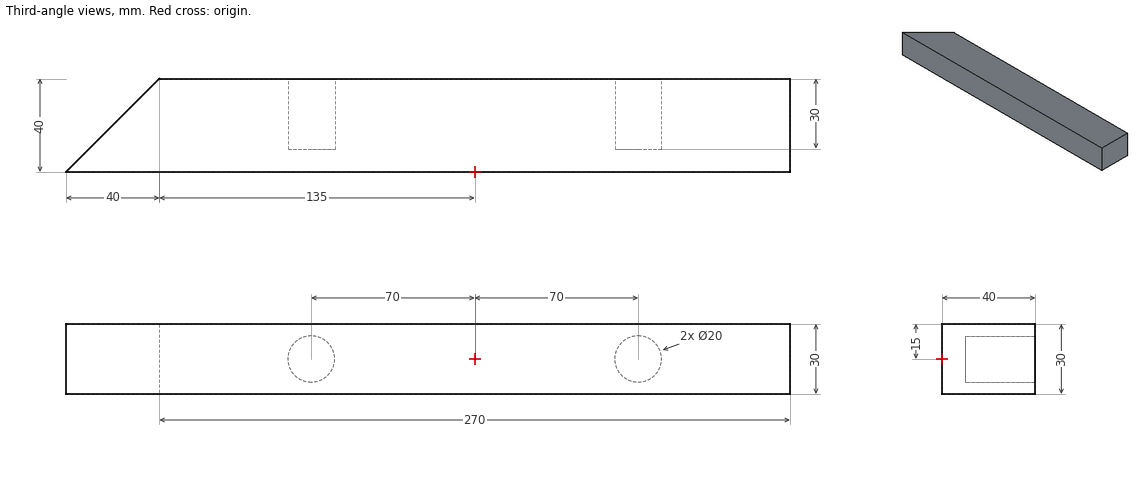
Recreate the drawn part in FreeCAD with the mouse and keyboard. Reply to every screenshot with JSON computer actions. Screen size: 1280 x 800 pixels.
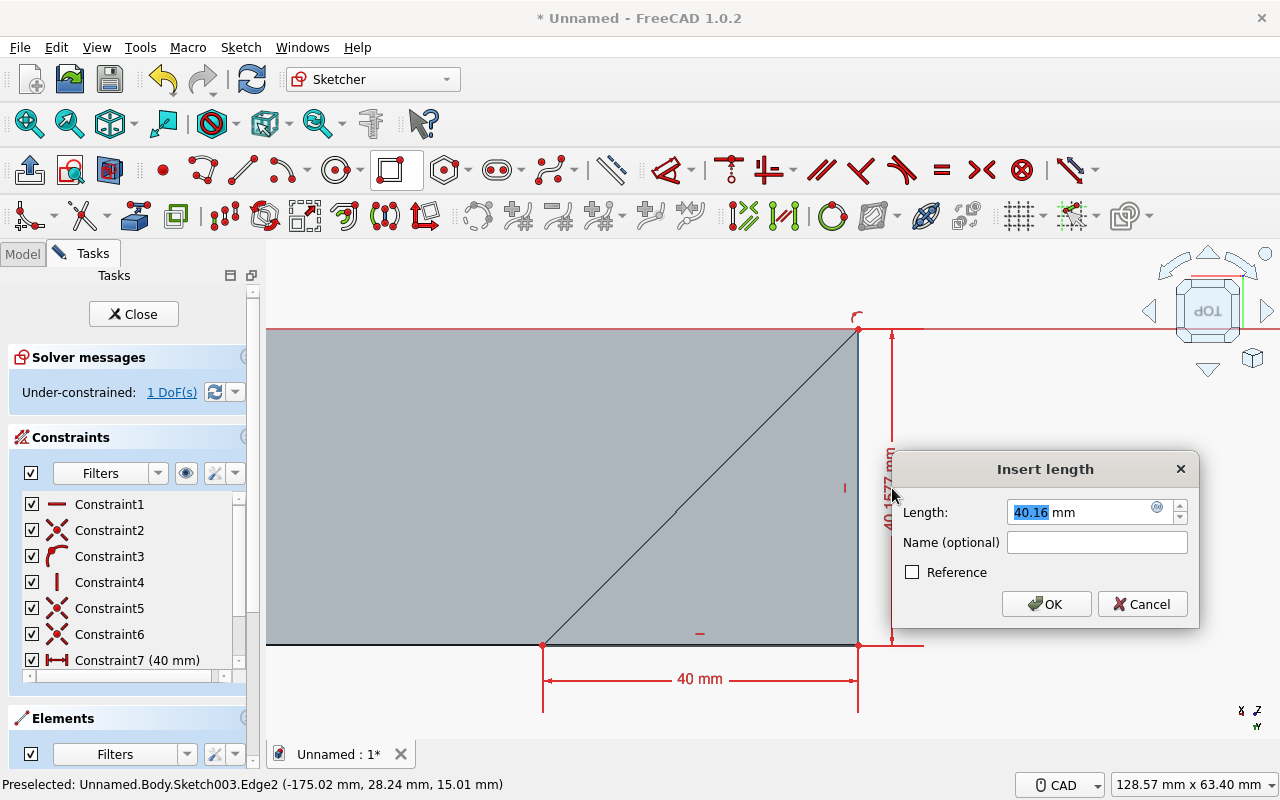
{"action": "type", "text": "40"}
{"action": "key", "text": "Return"}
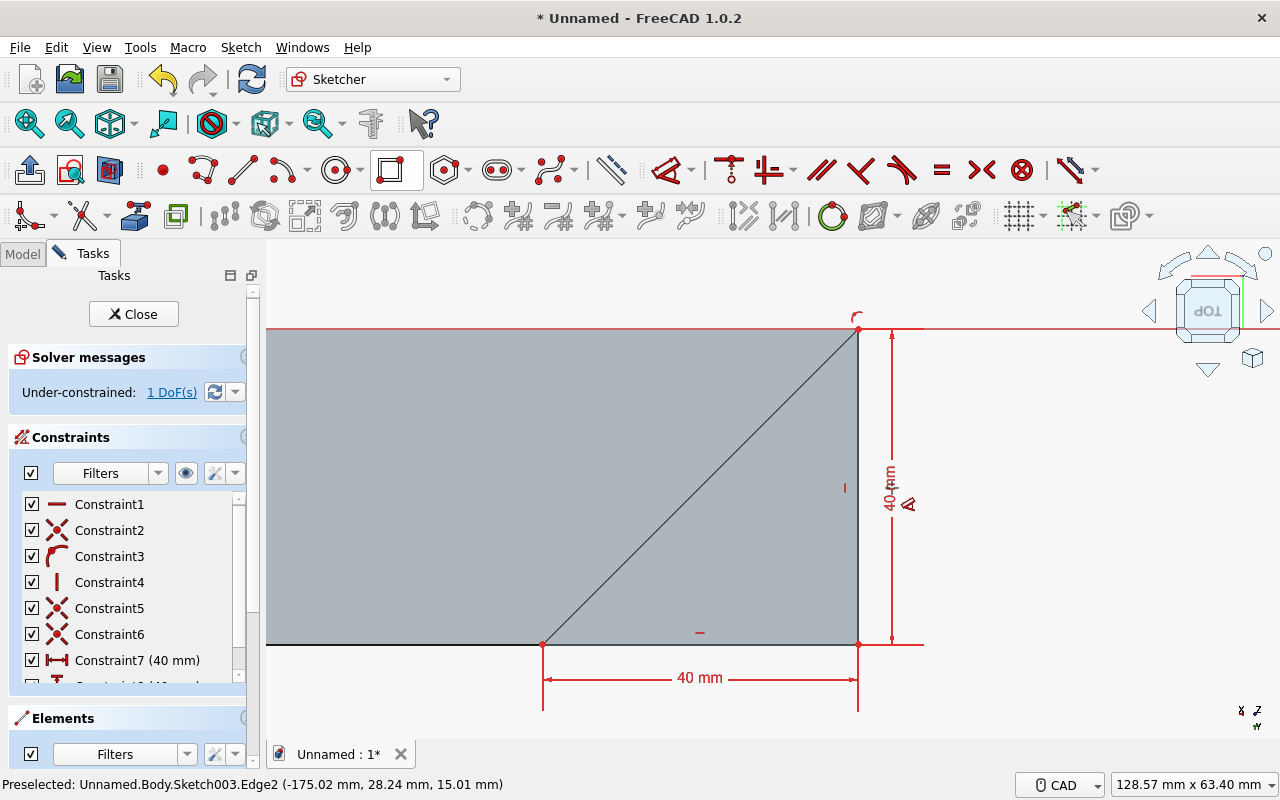
{"action": "left_click", "coordinate": [543, 645]}
{"action": "left_click", "coordinate": [418, 679]}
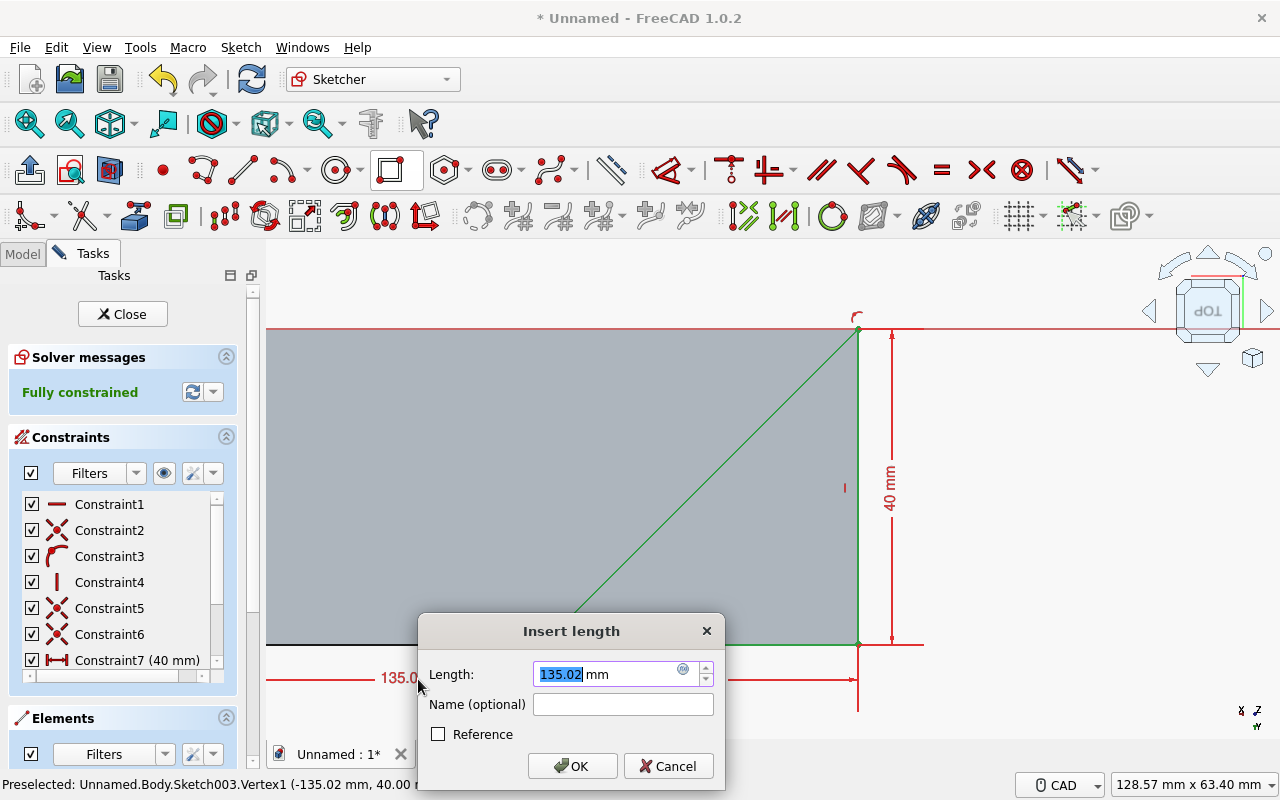
{"action": "type", "text": "135"}
{"action": "key", "text": "Return"}
{"action": "key", "text": "Escape"}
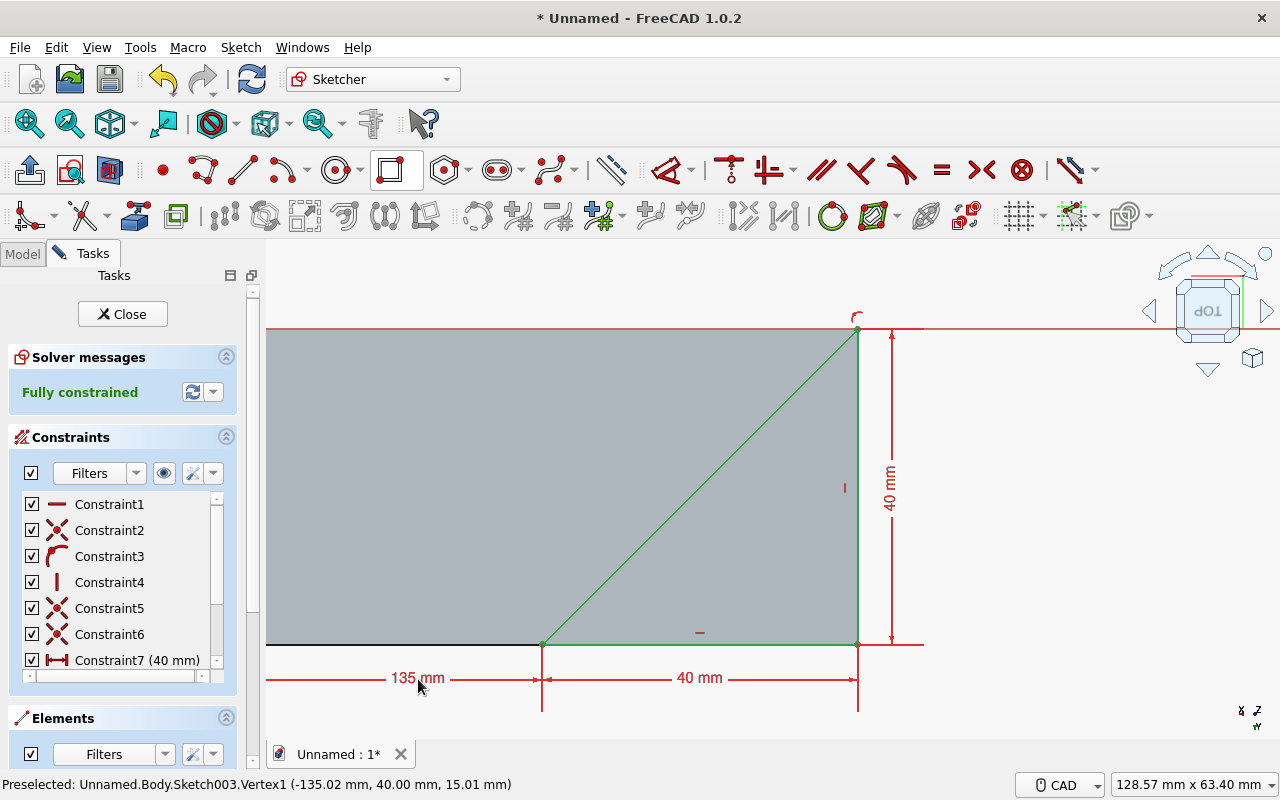
{"action": "left_click", "coordinate": [123, 314]}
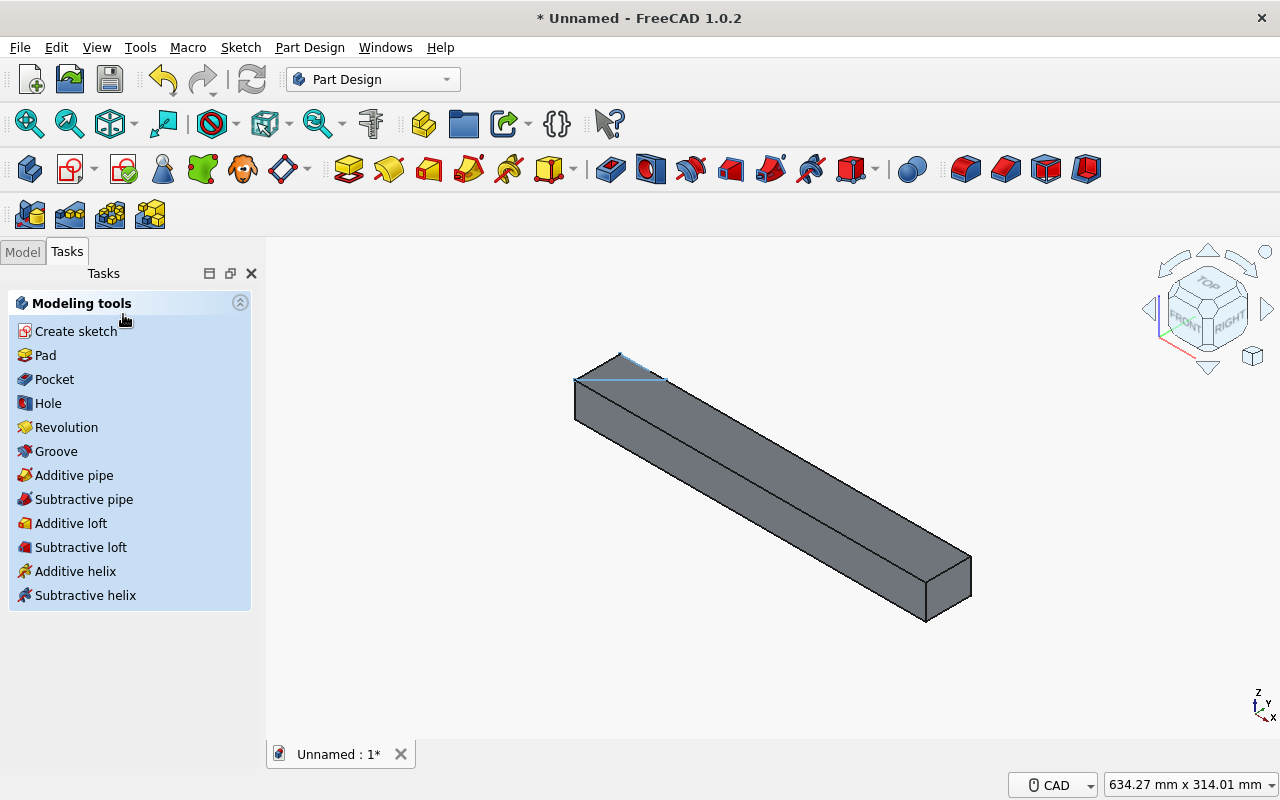
{"action": "left_click", "coordinate": [612, 170]}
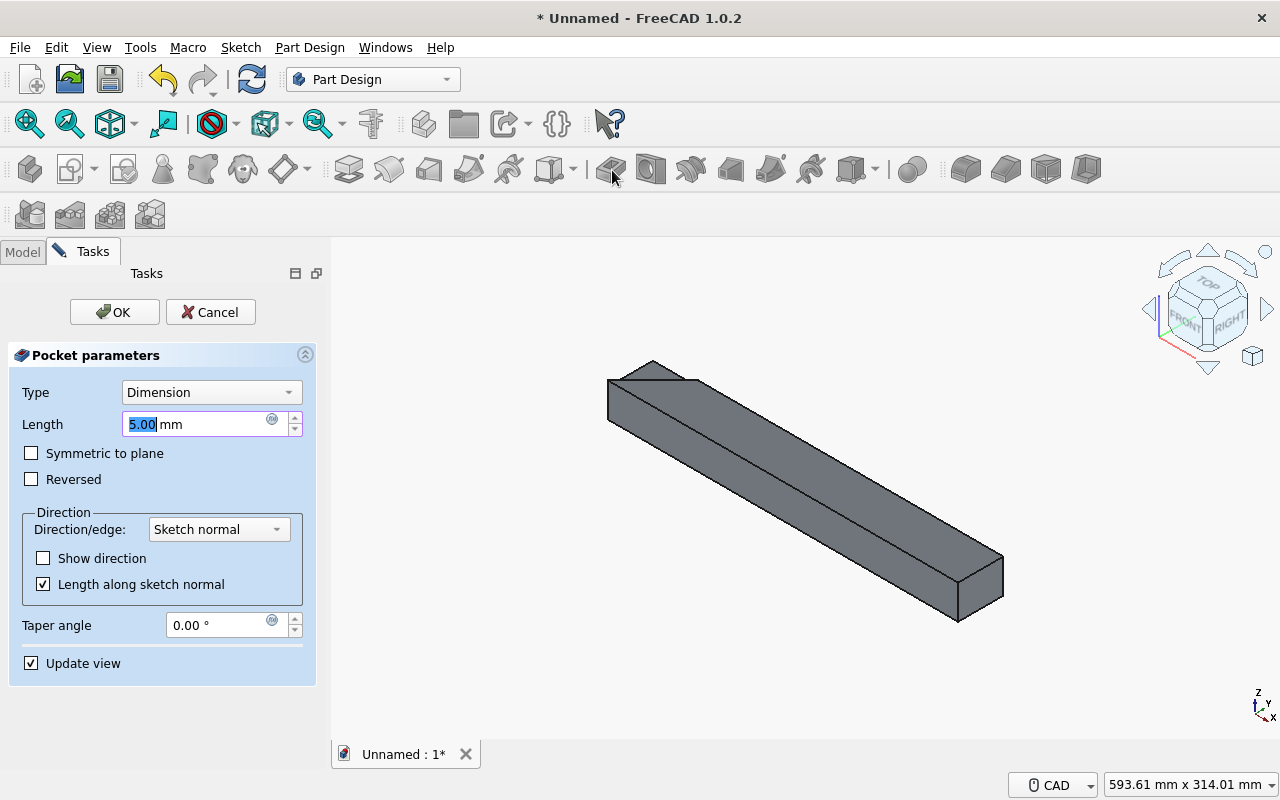
{"action": "left_click", "coordinate": [212, 392]}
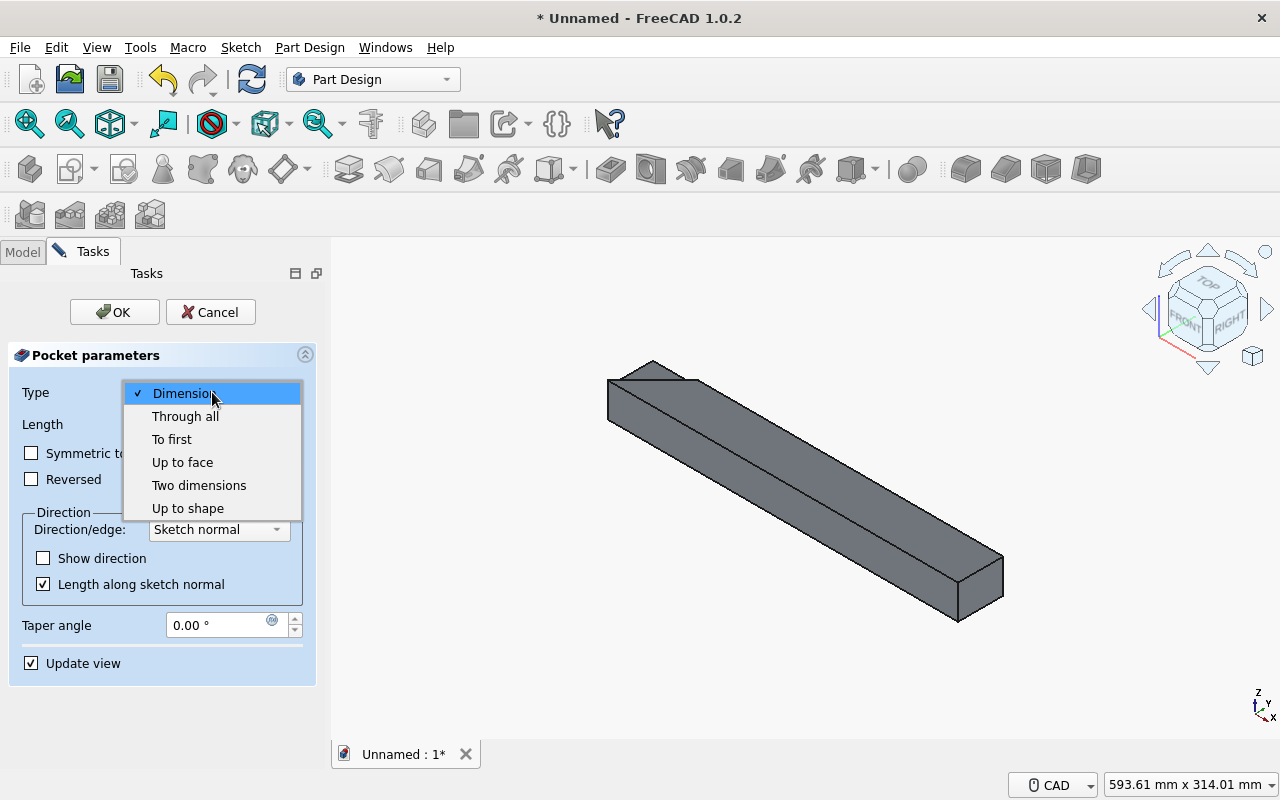
{"action": "left_click", "coordinate": [212, 416]}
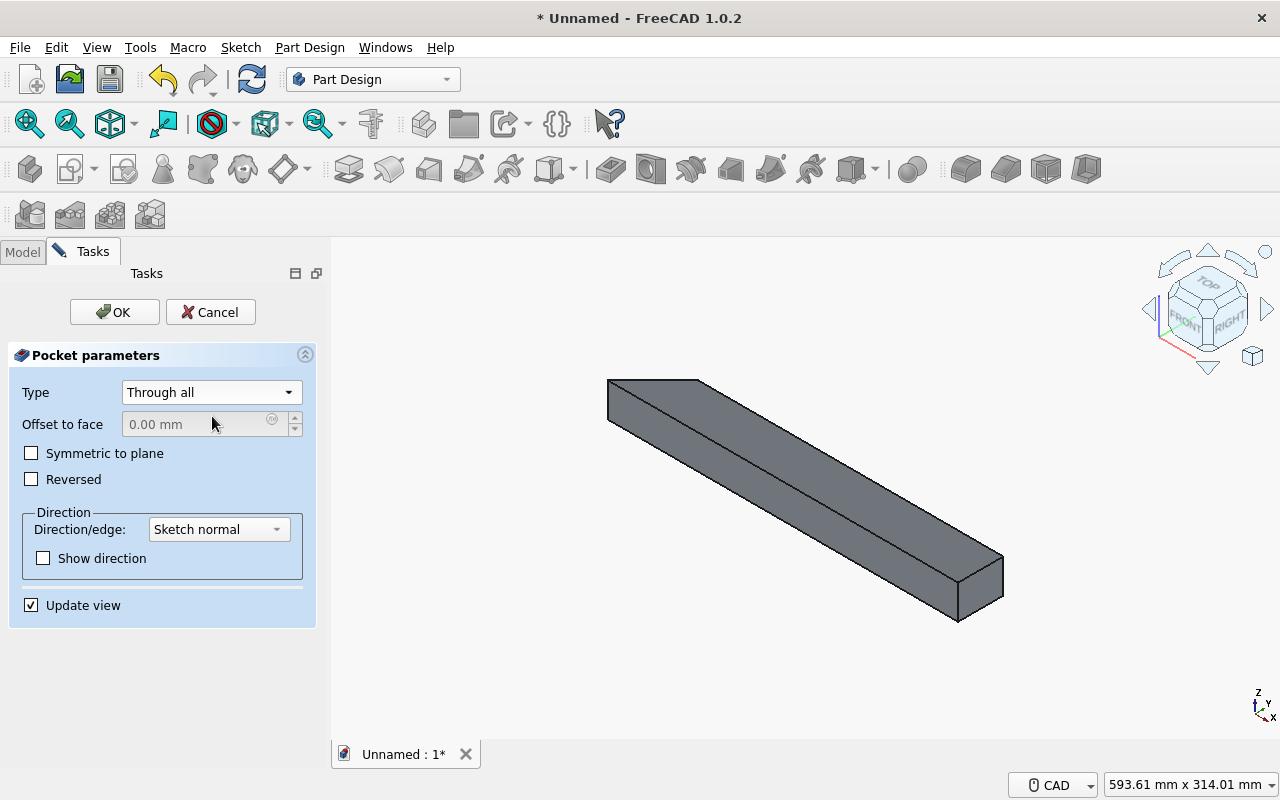
{"action": "left_click", "coordinate": [115, 312]}